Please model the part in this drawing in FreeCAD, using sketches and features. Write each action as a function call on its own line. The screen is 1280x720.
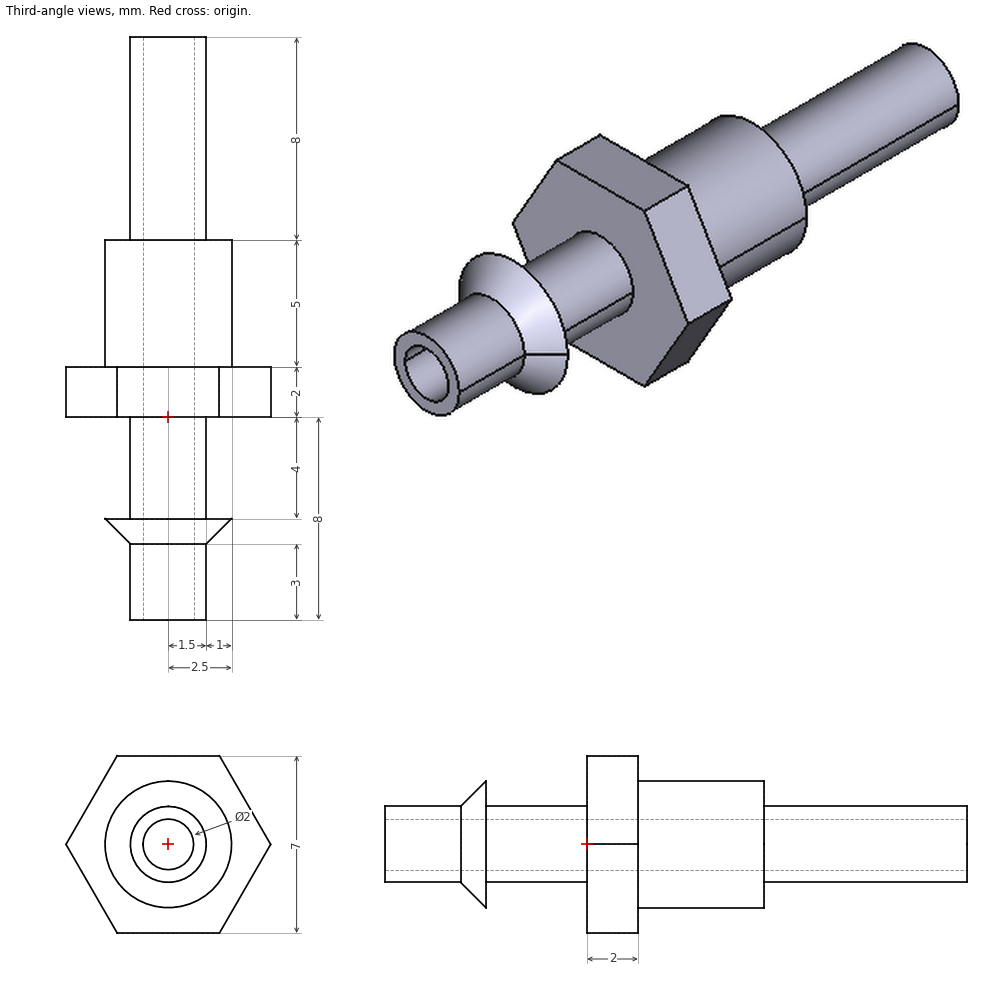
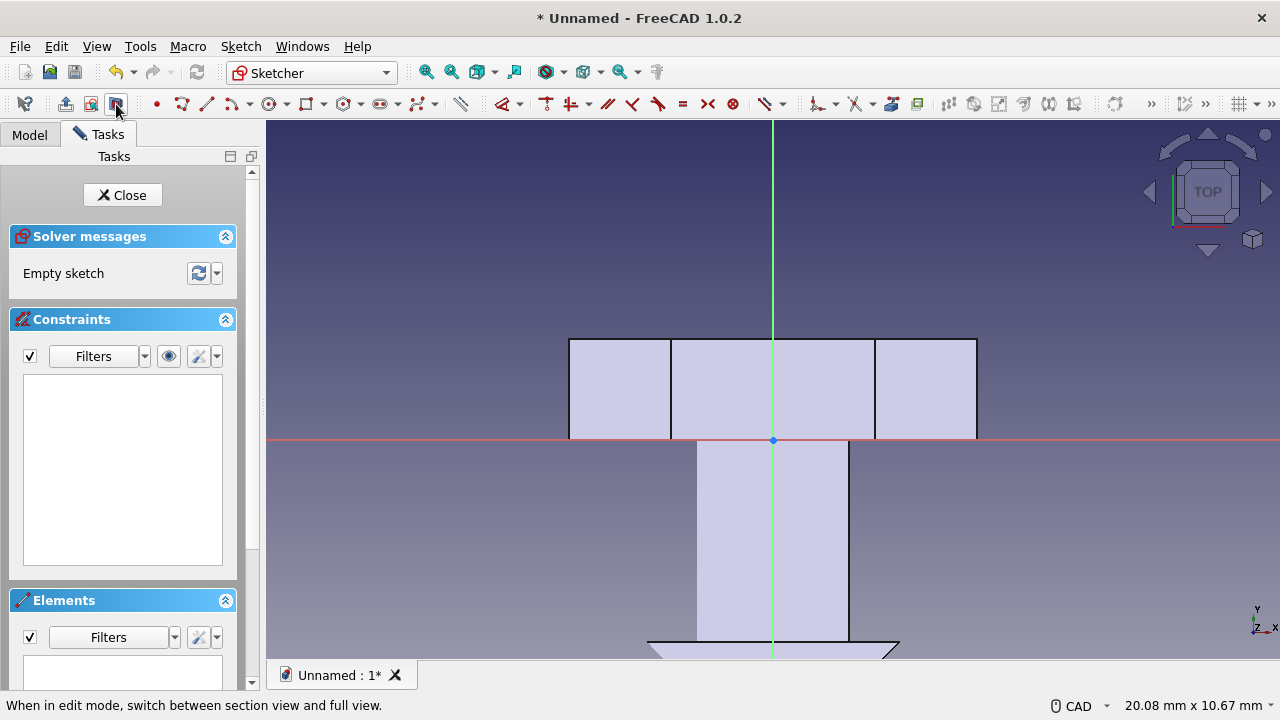
scroll(597, 631, down, 4)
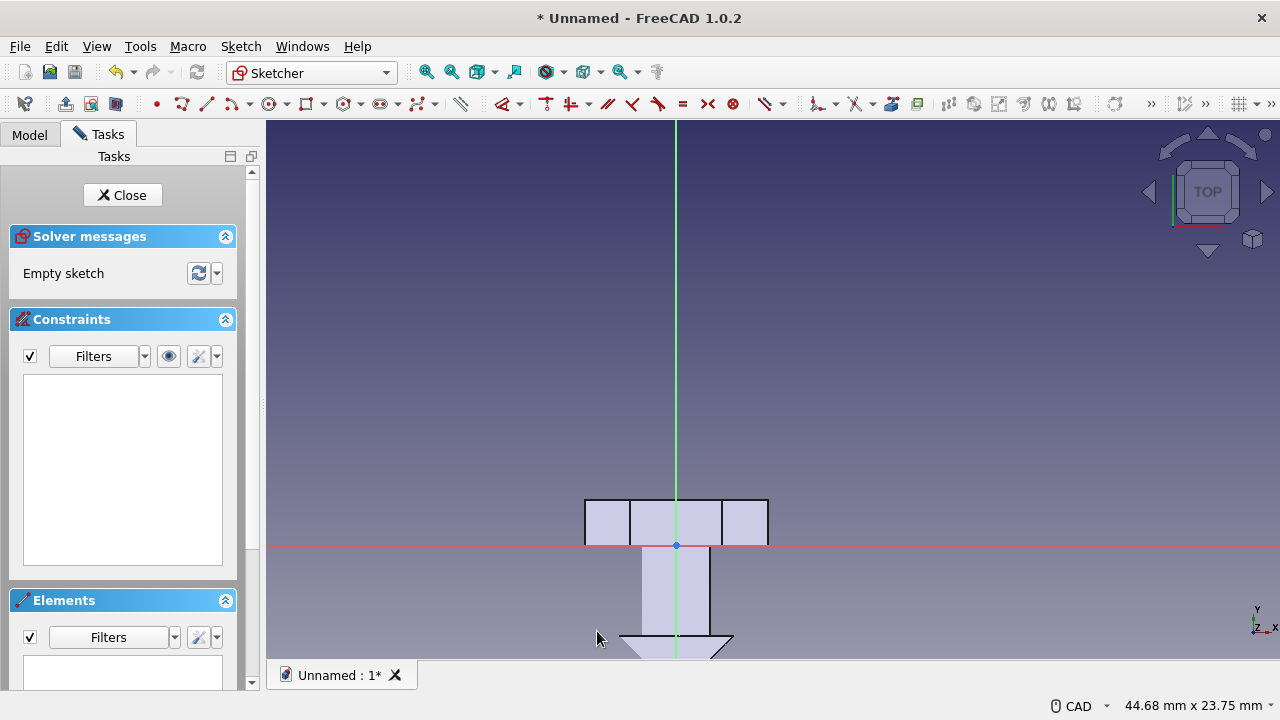
click(182, 104)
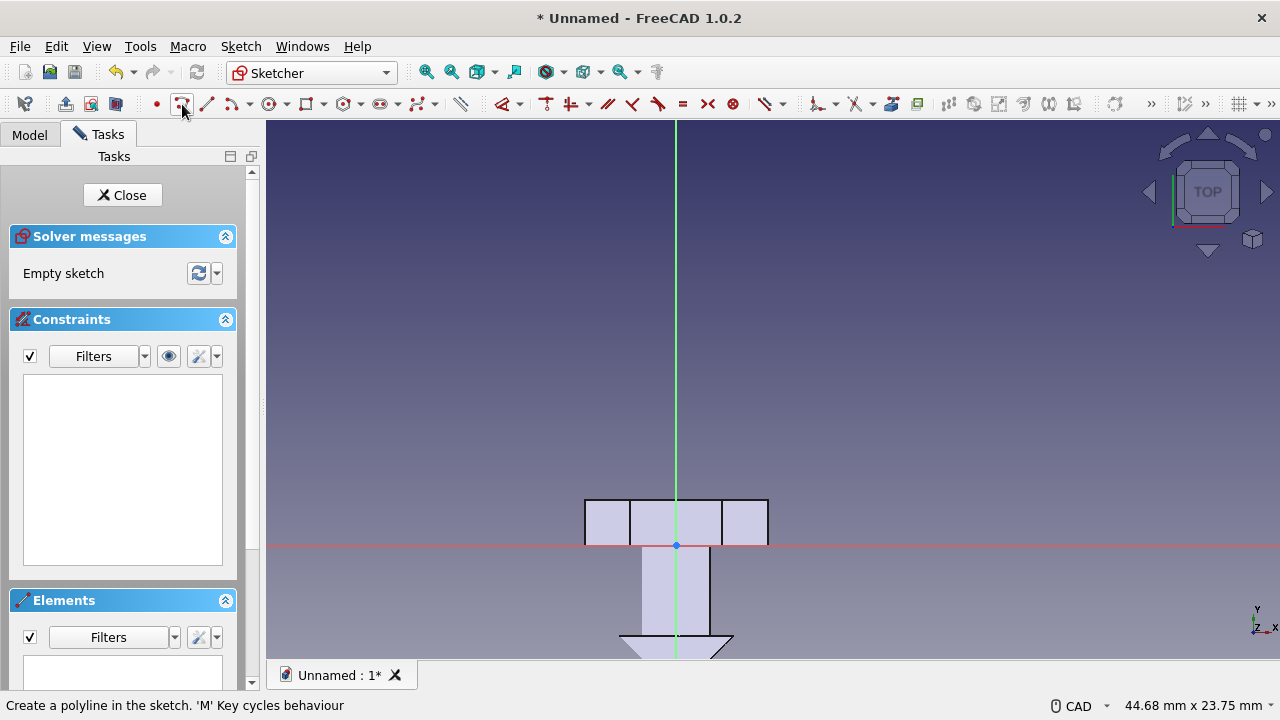
click(676, 500)
click(733, 500)
click(733, 387)
click(710, 387)
click(710, 205)
click(685, 205)
click(676, 501)
key(Escape)
key(Escape)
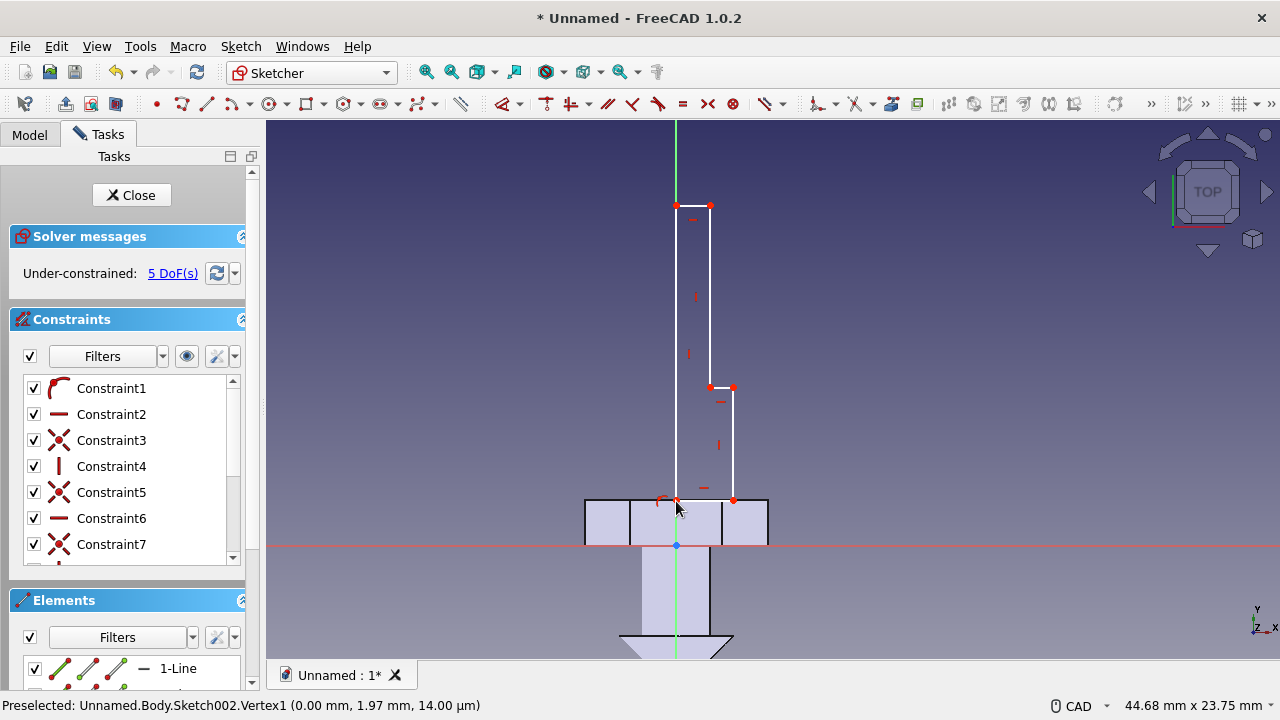
key(d)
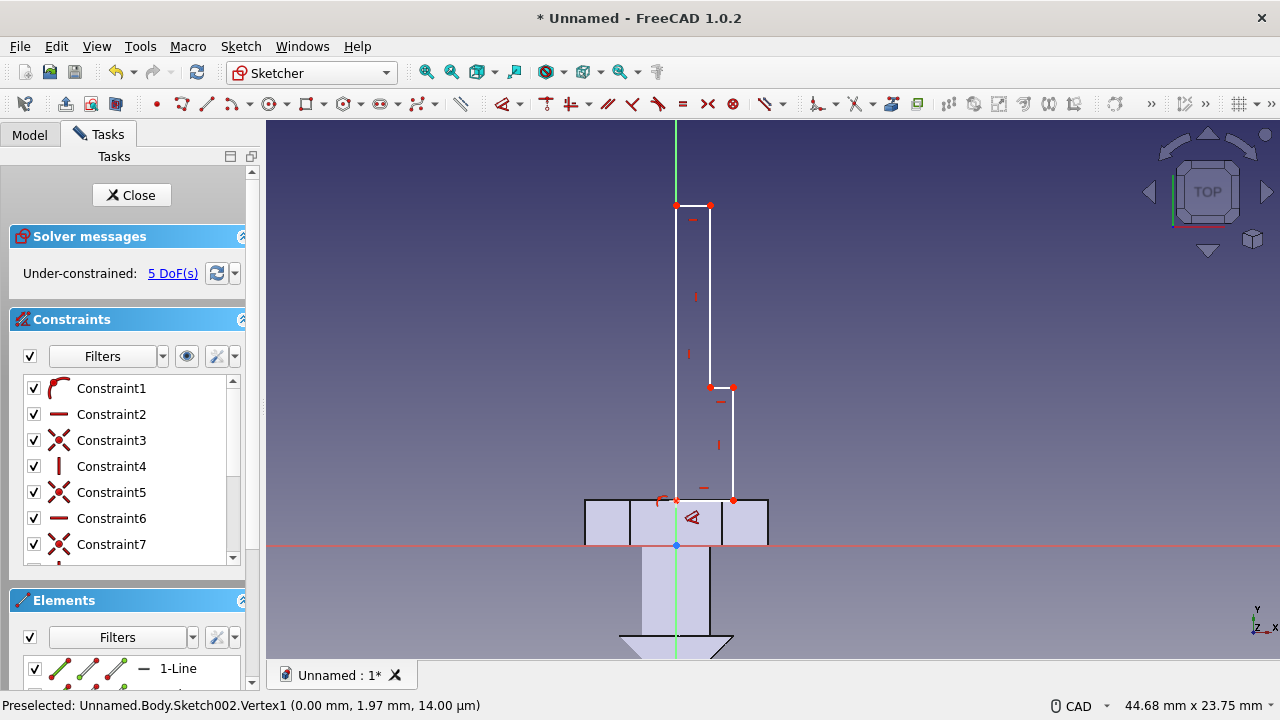
click(733, 467)
click(767, 444)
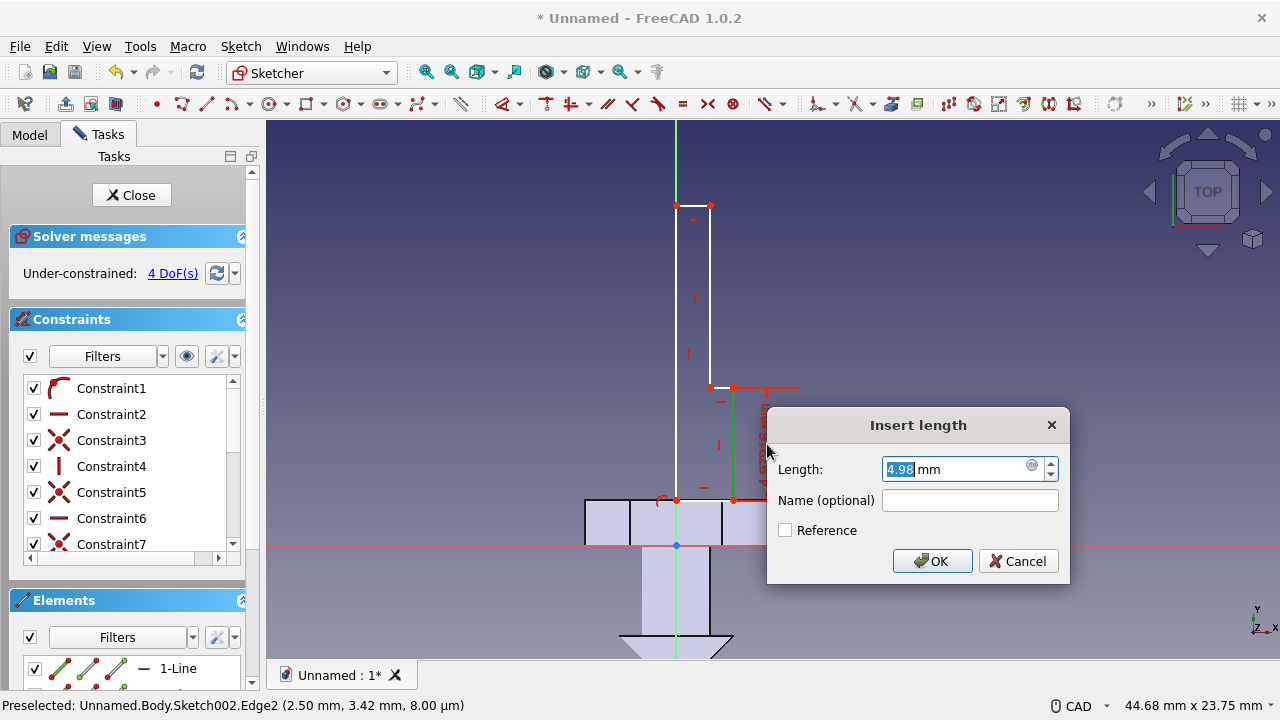
text(5)
key(Return)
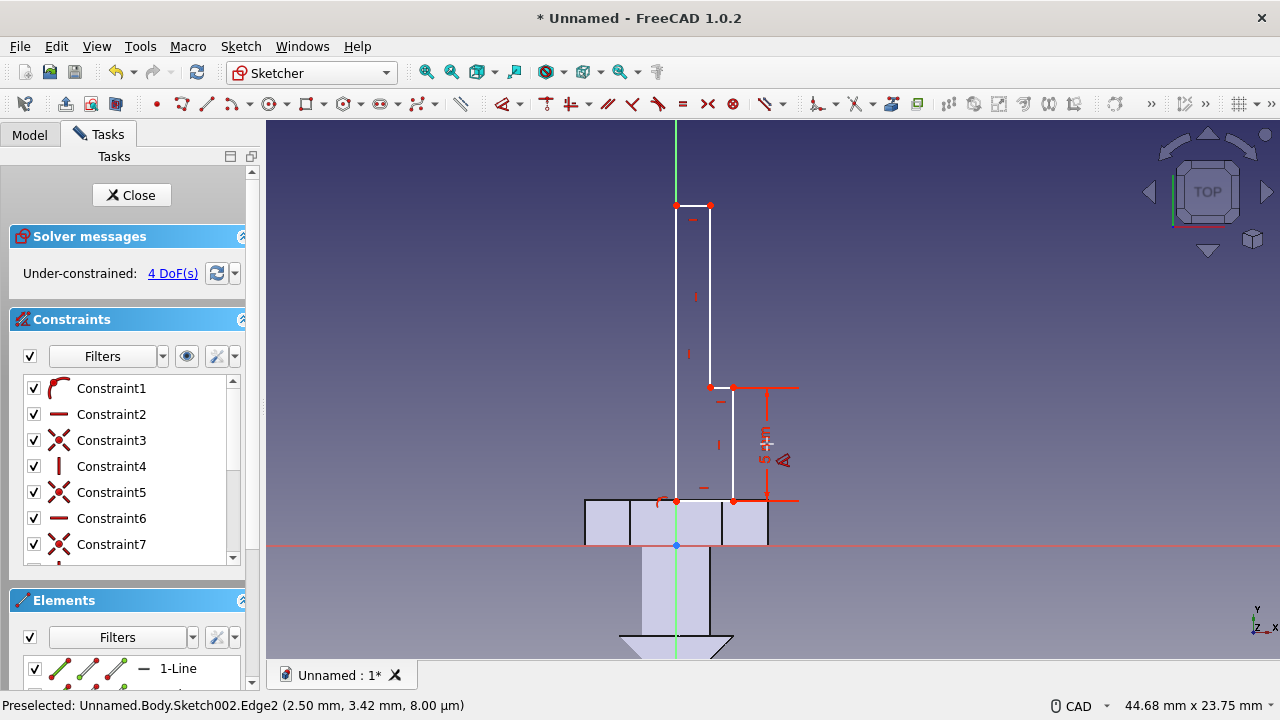
scroll(724, 388, up, 3)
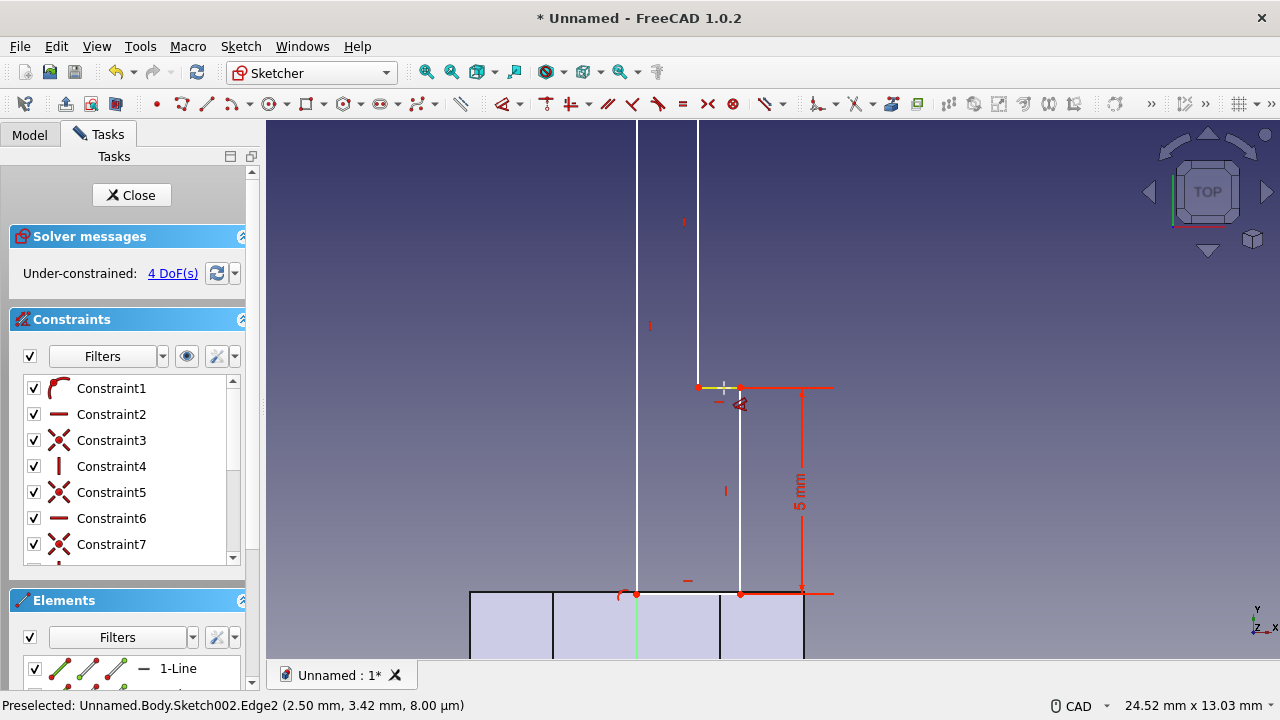
click(723, 388)
click(719, 422)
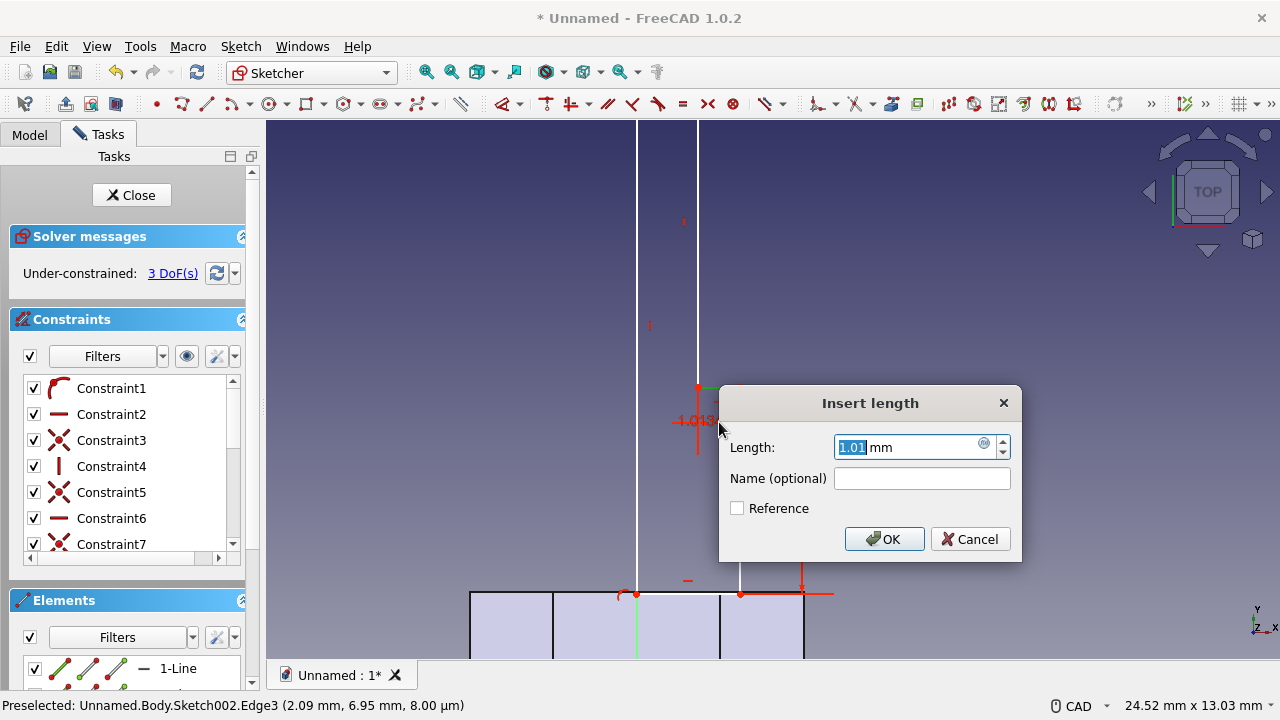
text(1)
key(Return)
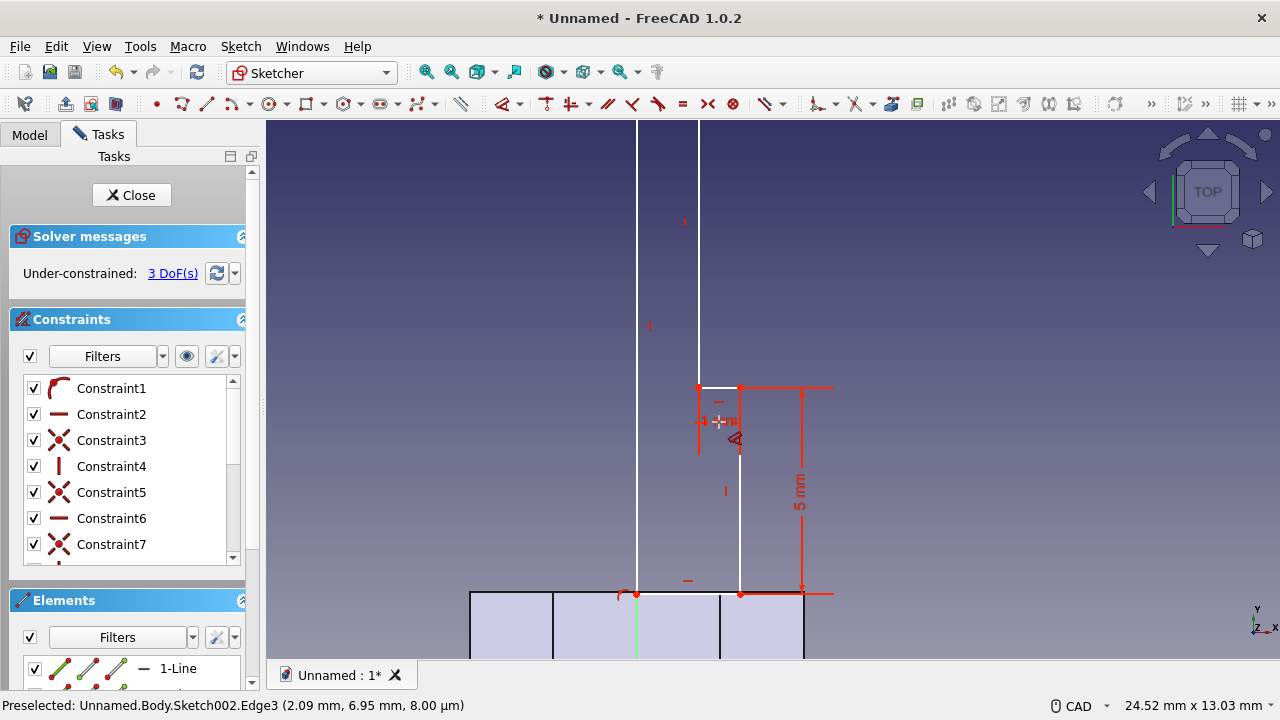
click(699, 288)
click(733, 268)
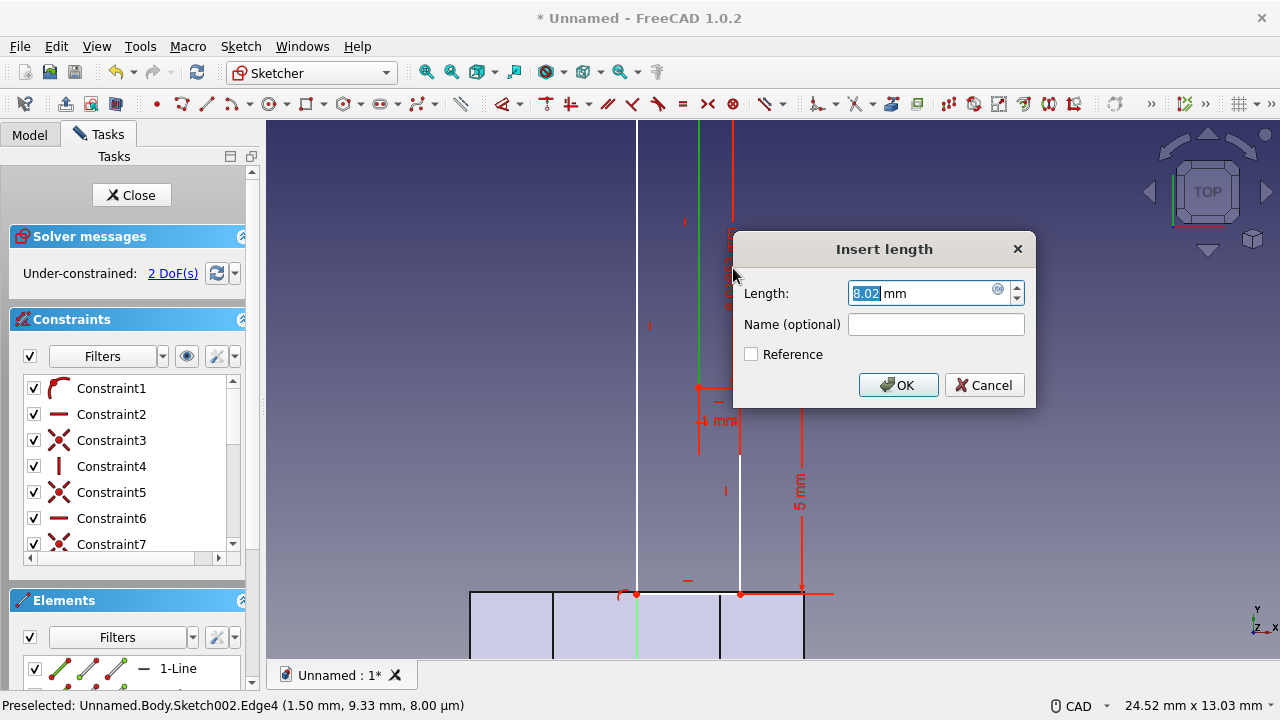
text(8)
key(Return)